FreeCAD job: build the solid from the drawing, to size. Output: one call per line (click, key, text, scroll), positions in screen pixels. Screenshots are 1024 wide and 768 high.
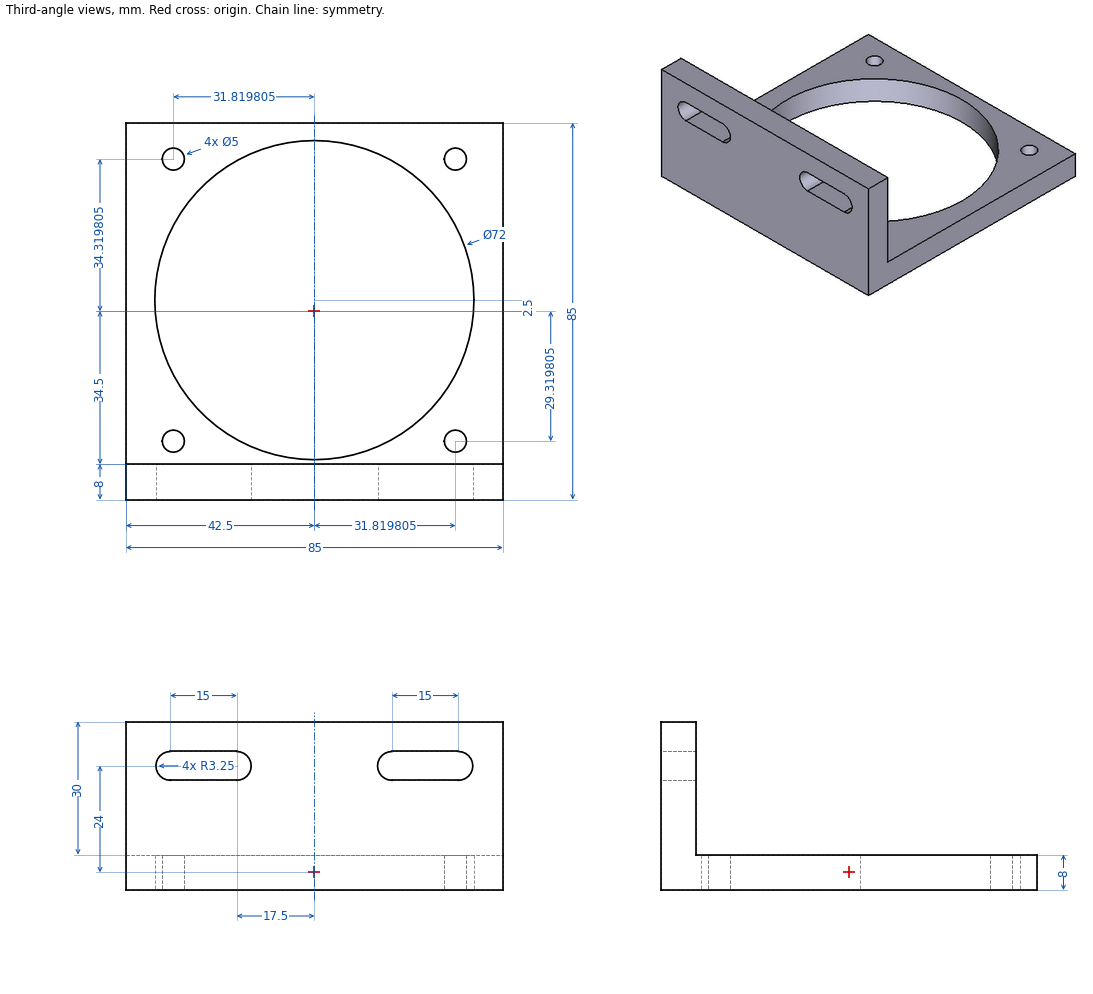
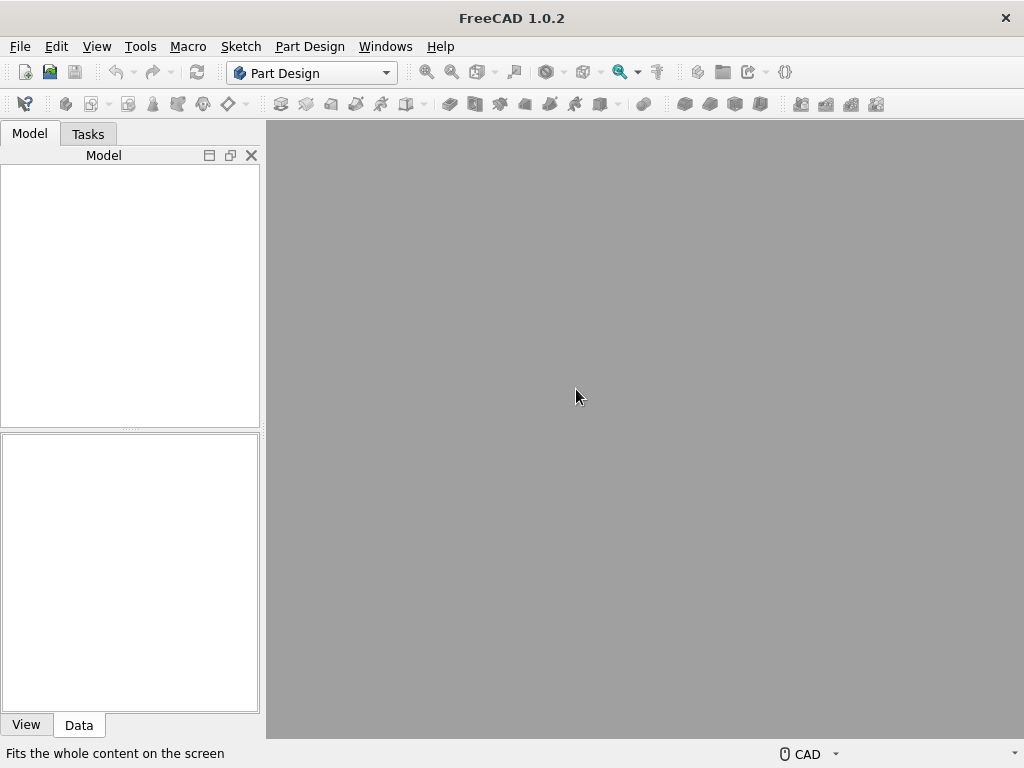
click(25, 72)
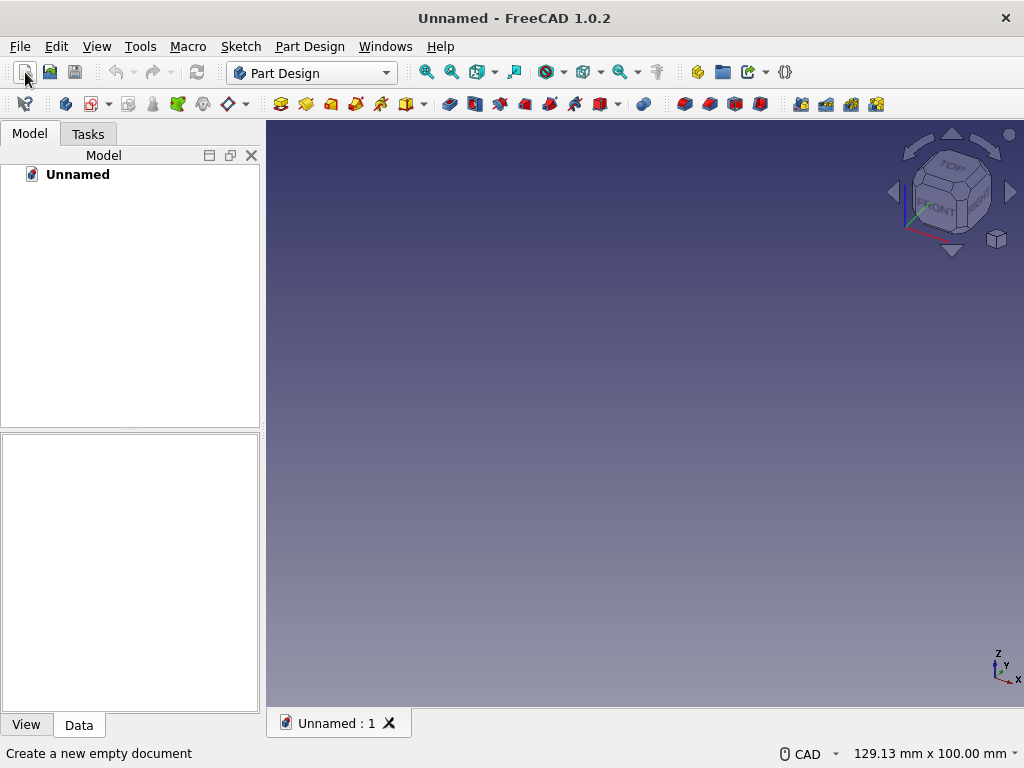
click(90, 104)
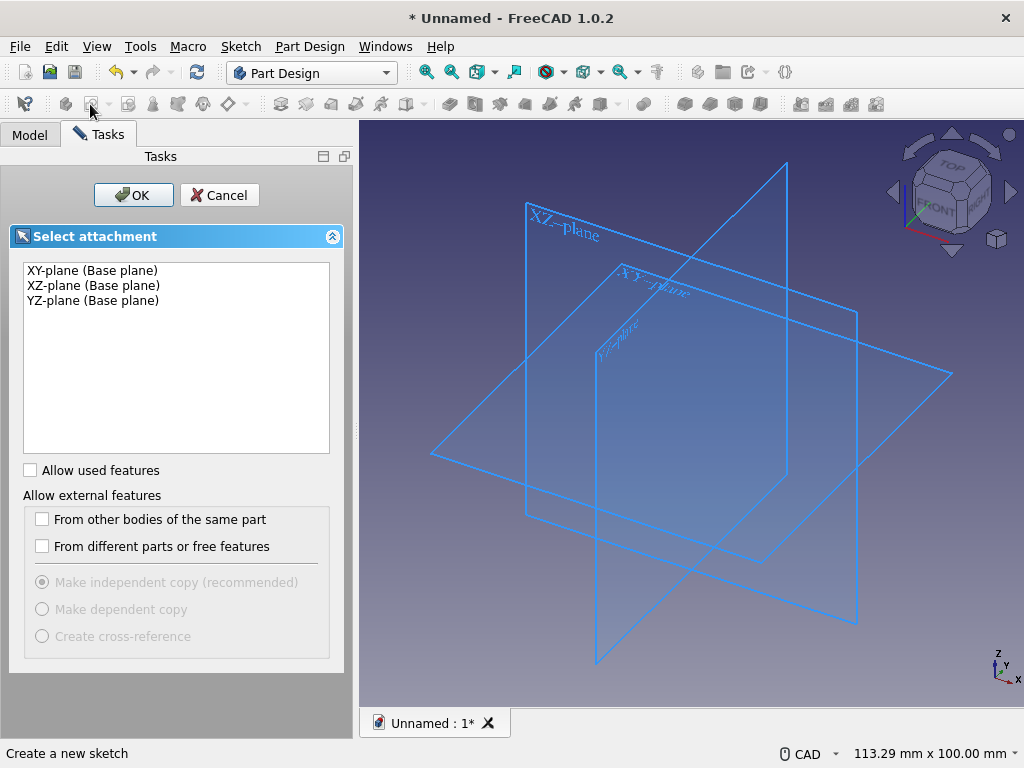
click(84, 270)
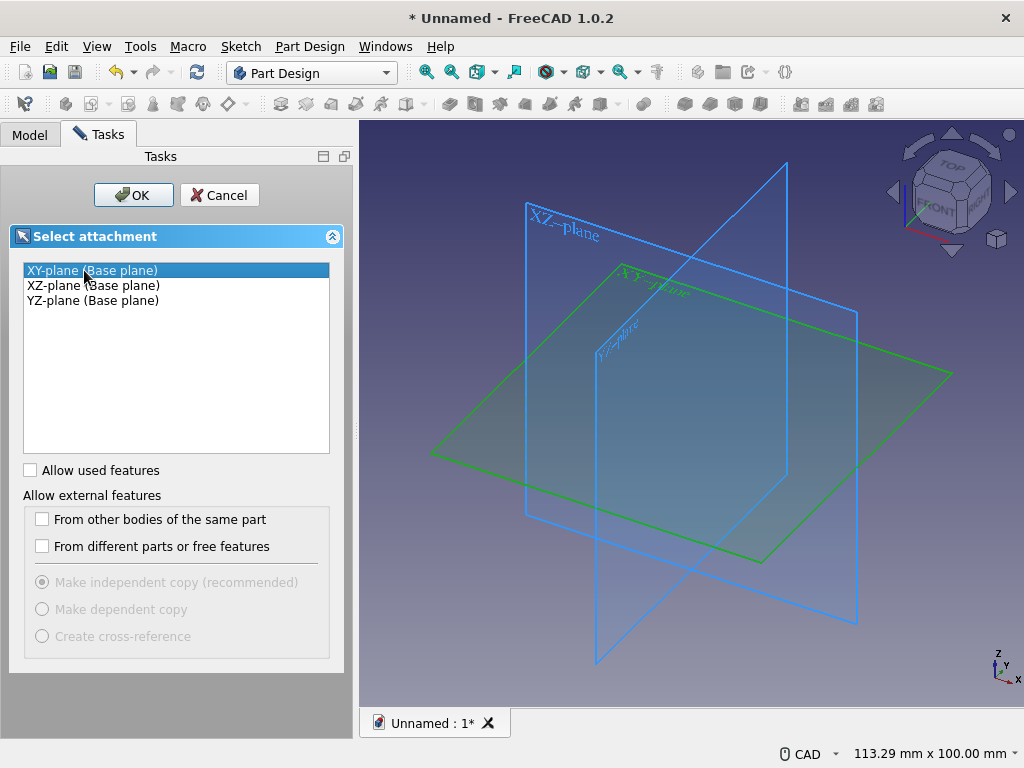
click(134, 195)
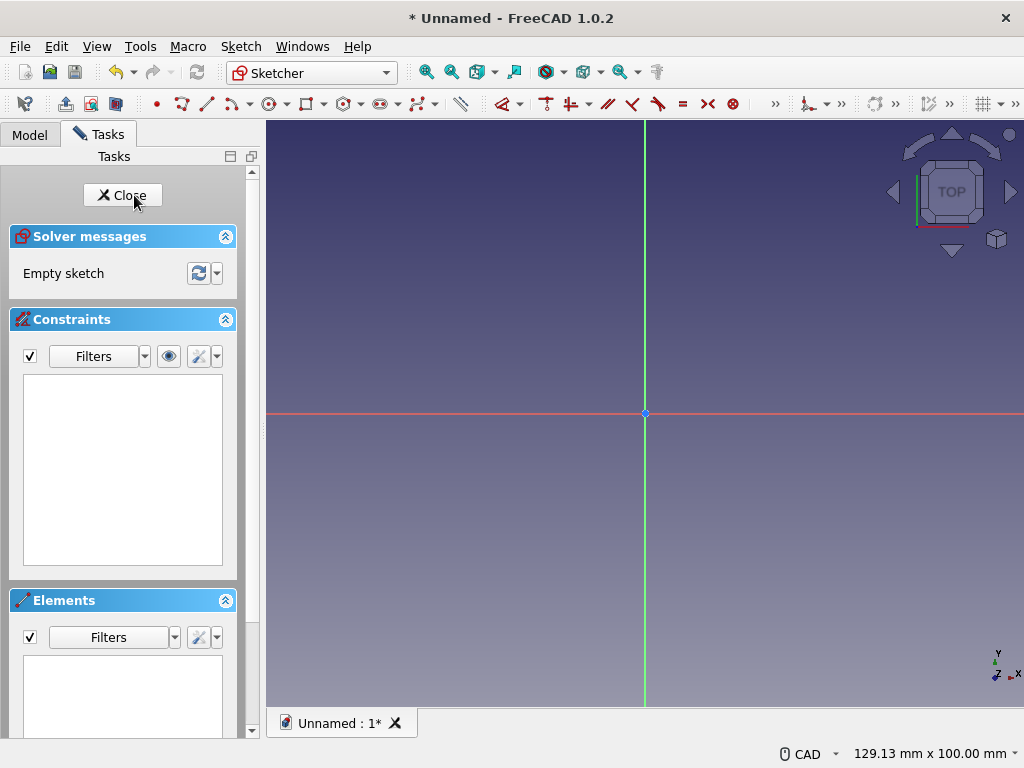
scroll(294, 413, down, 1)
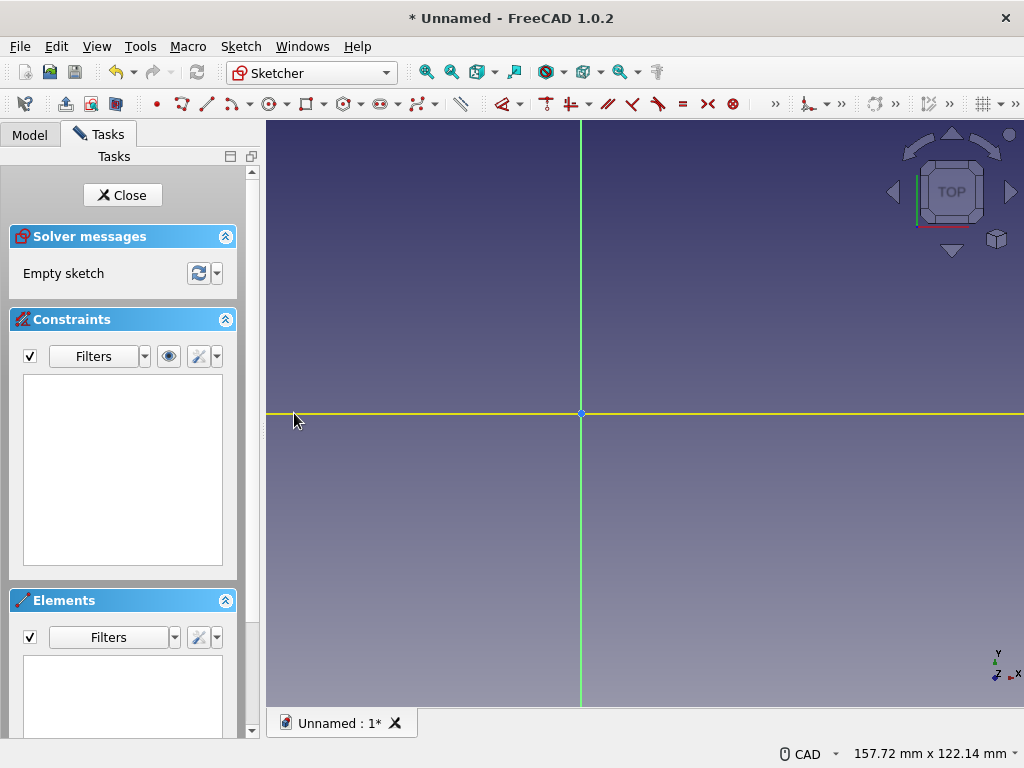
key(g)
key(v)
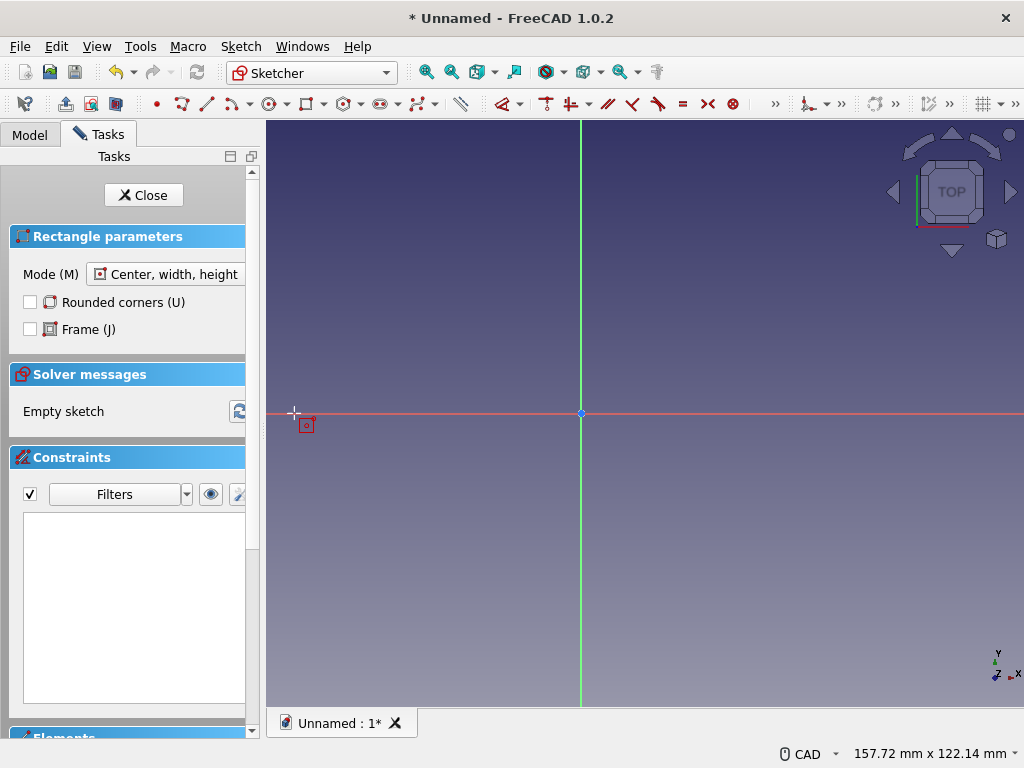
click(581, 414)
click(786, 209)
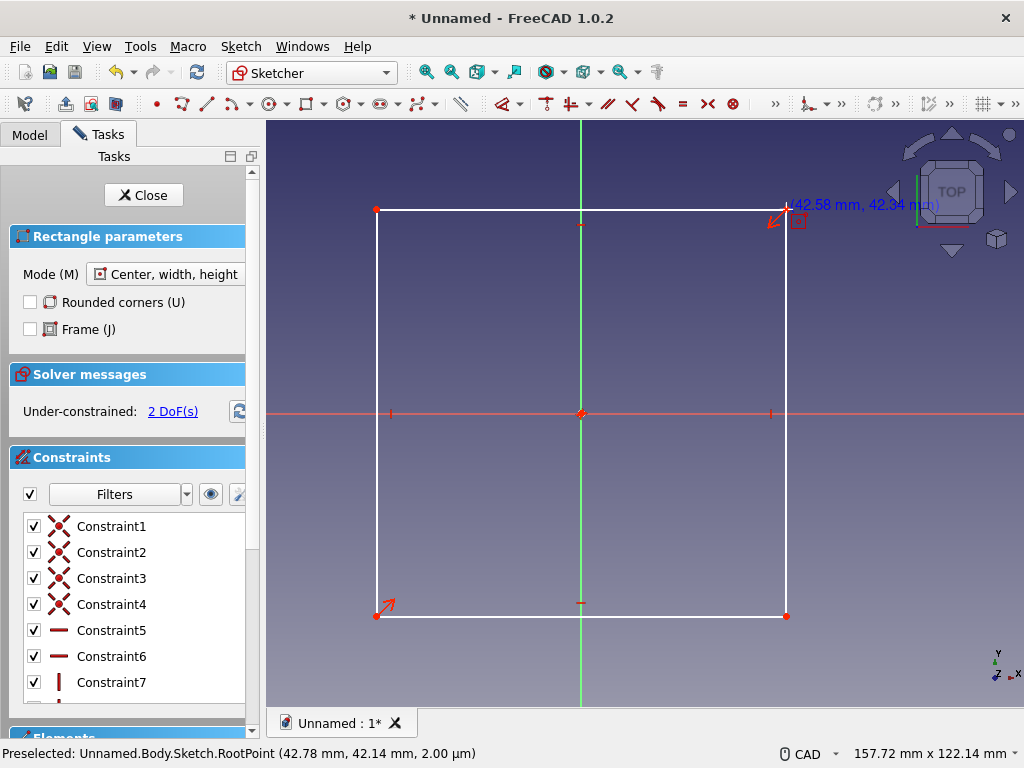
key(g)
key(c)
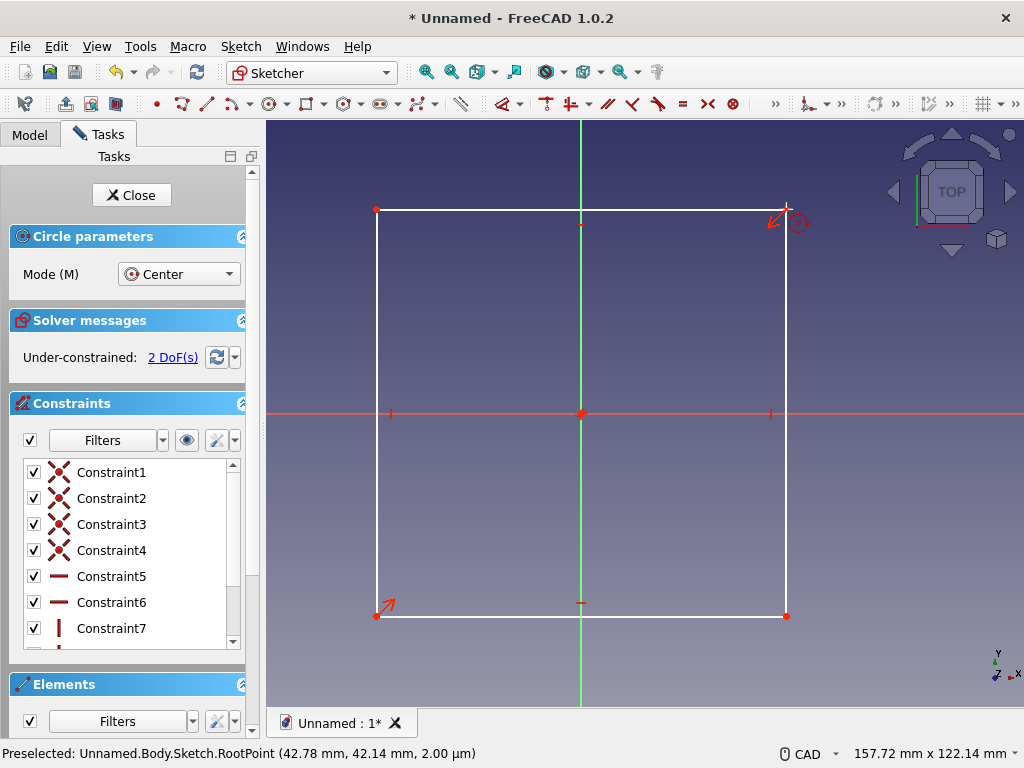
scroll(581, 401, up, 2)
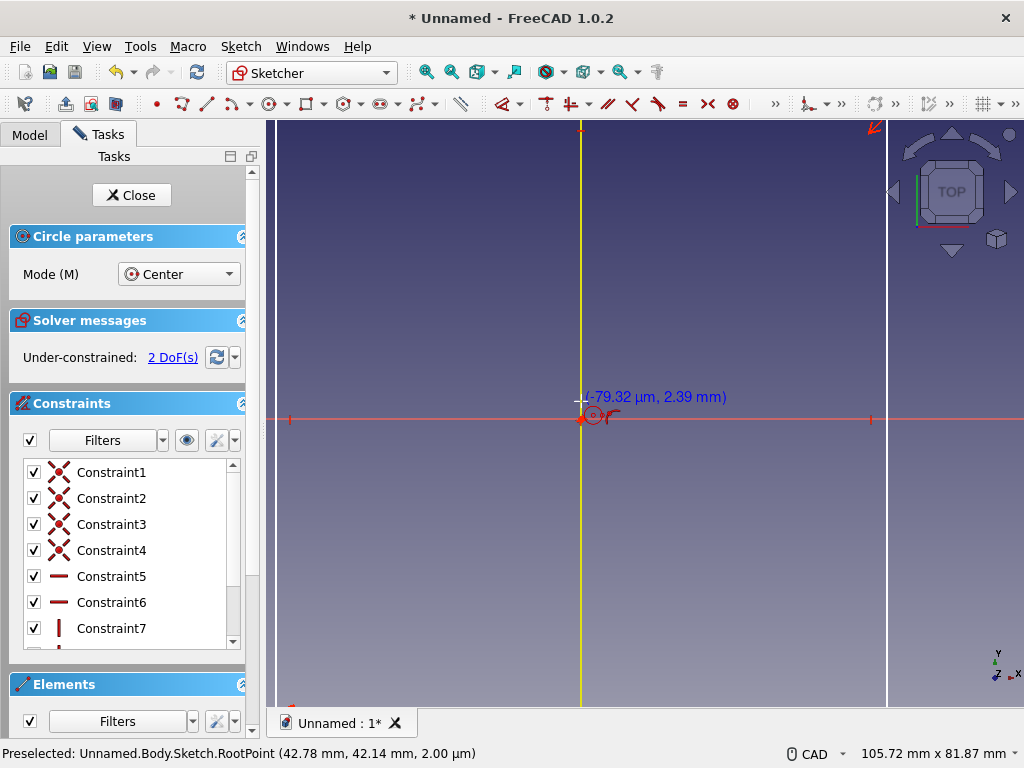
click(581, 401)
click(764, 219)
key(Escape)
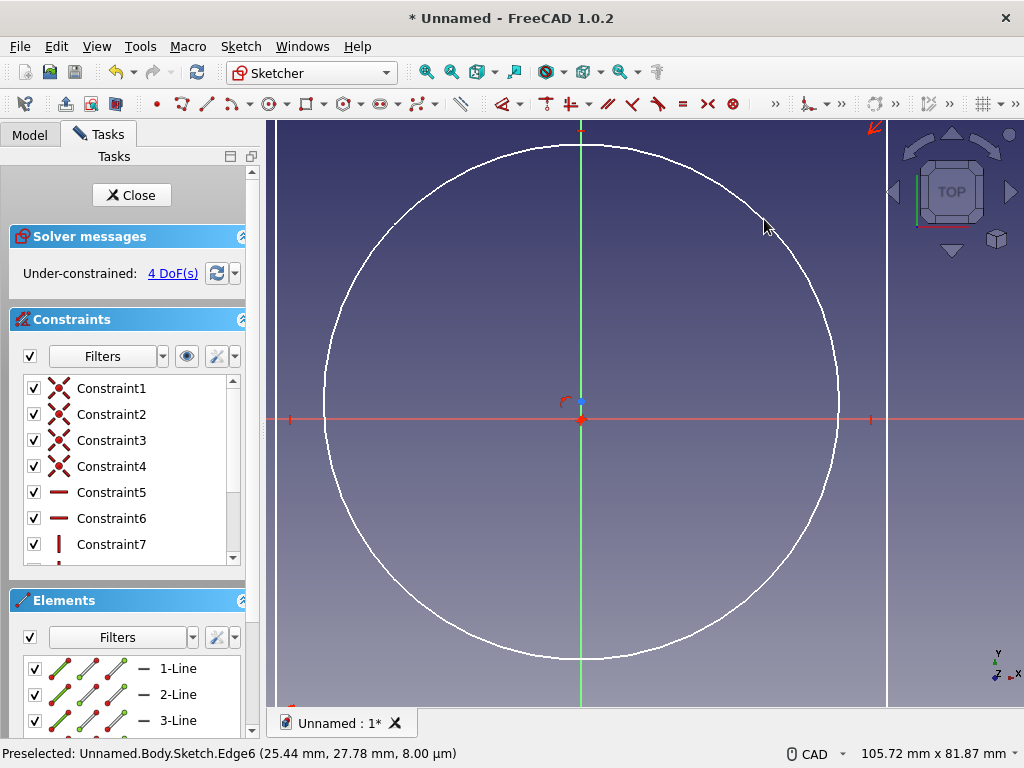
click(502, 104)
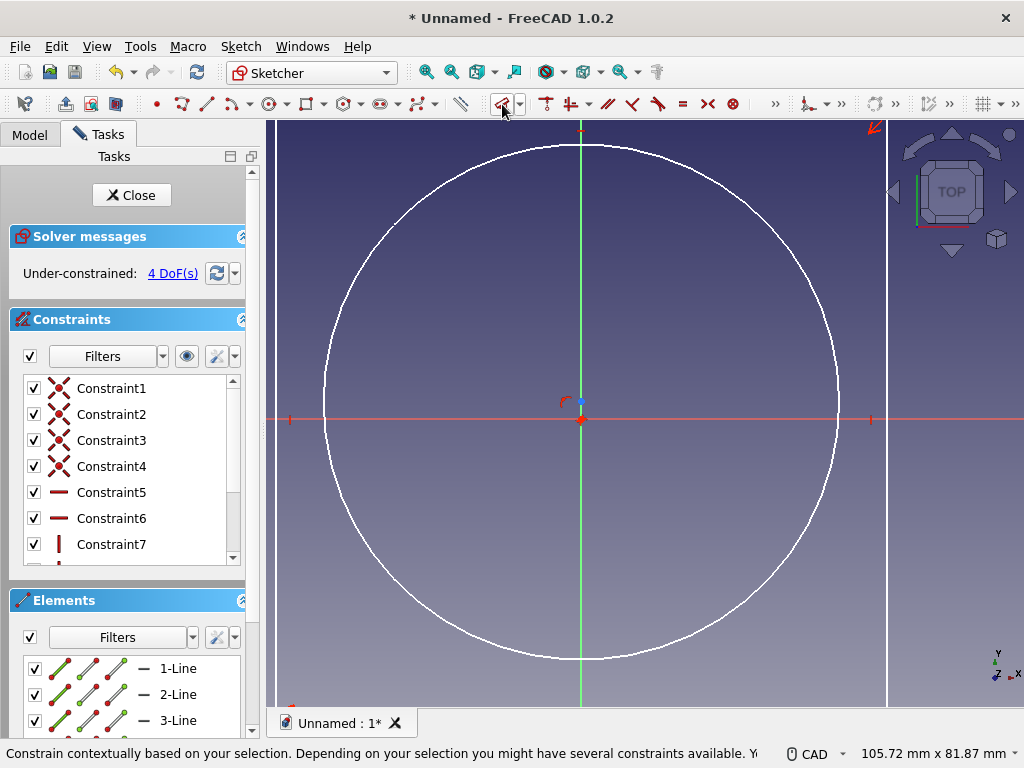
click(763, 219)
click(786, 196)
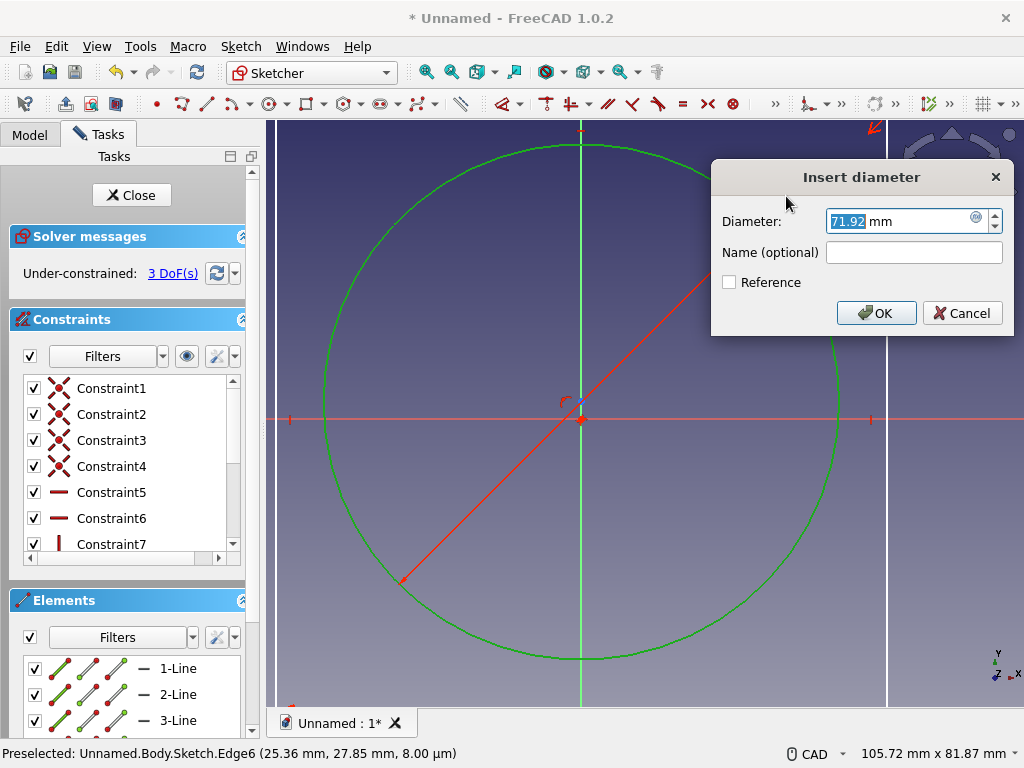
text(72)
key(Return)